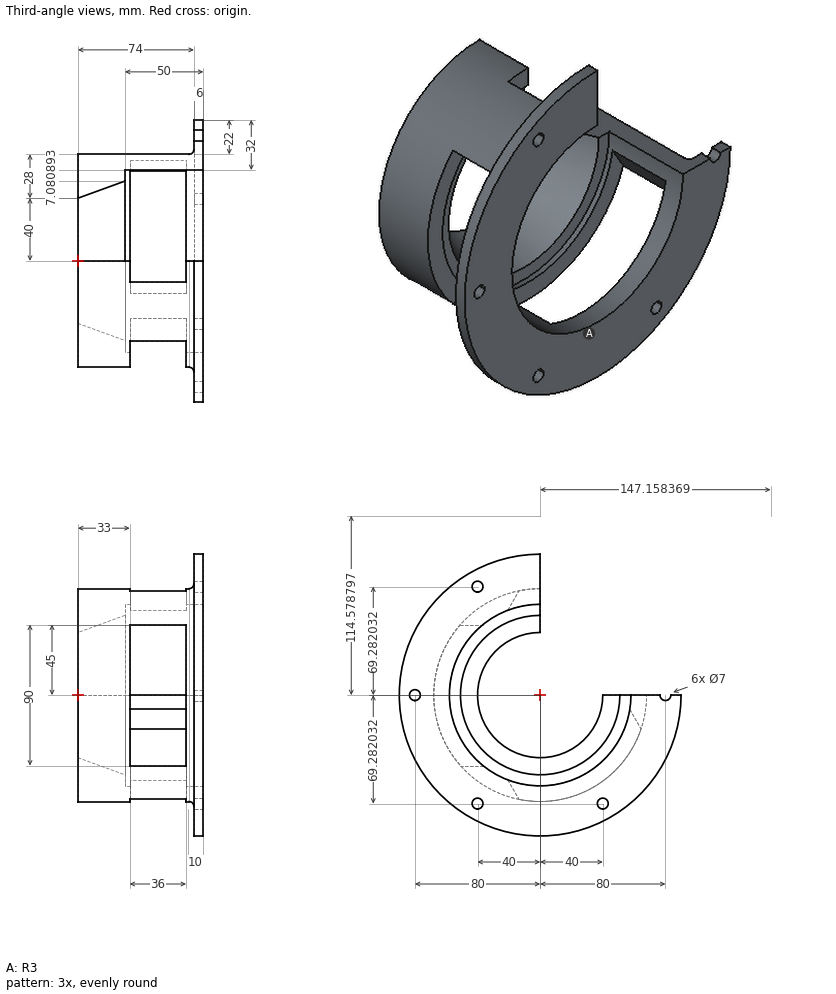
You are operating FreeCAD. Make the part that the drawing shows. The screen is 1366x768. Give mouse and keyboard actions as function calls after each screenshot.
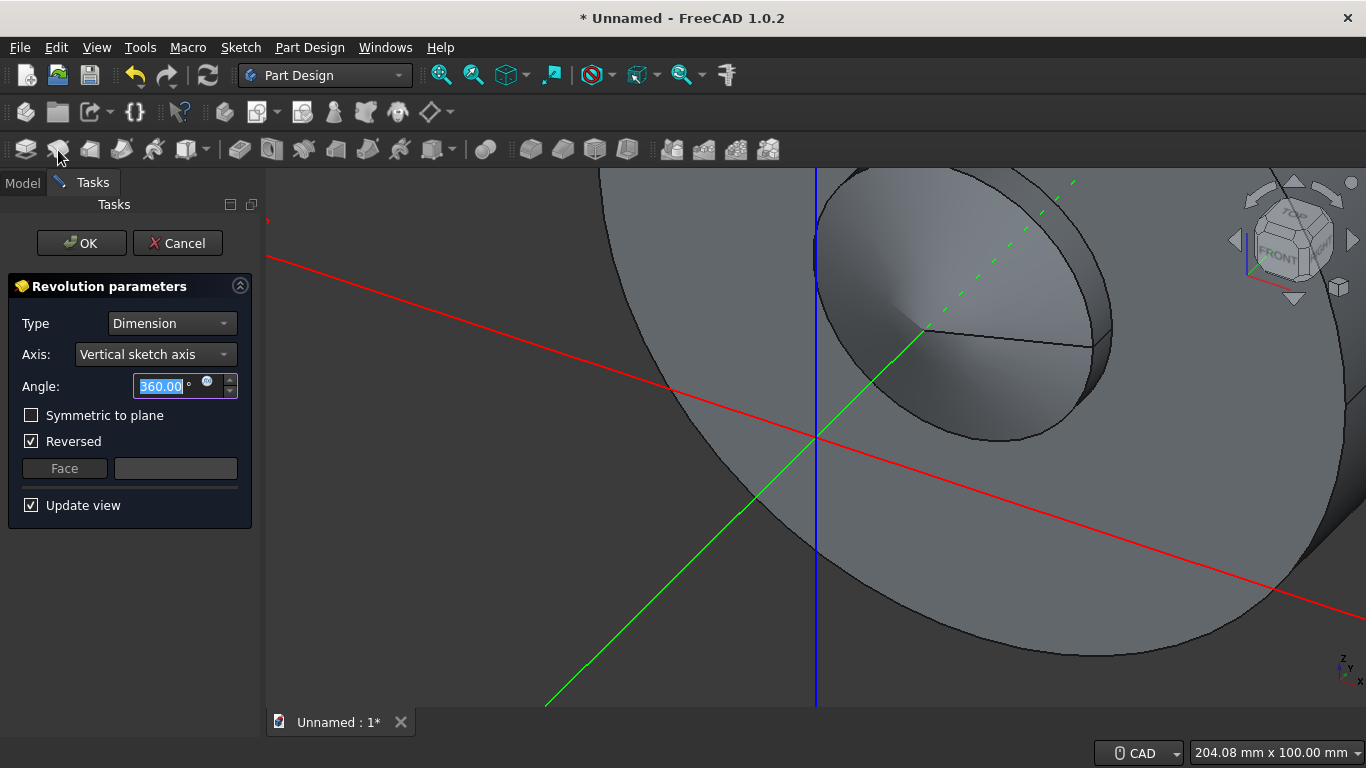
click(156, 354)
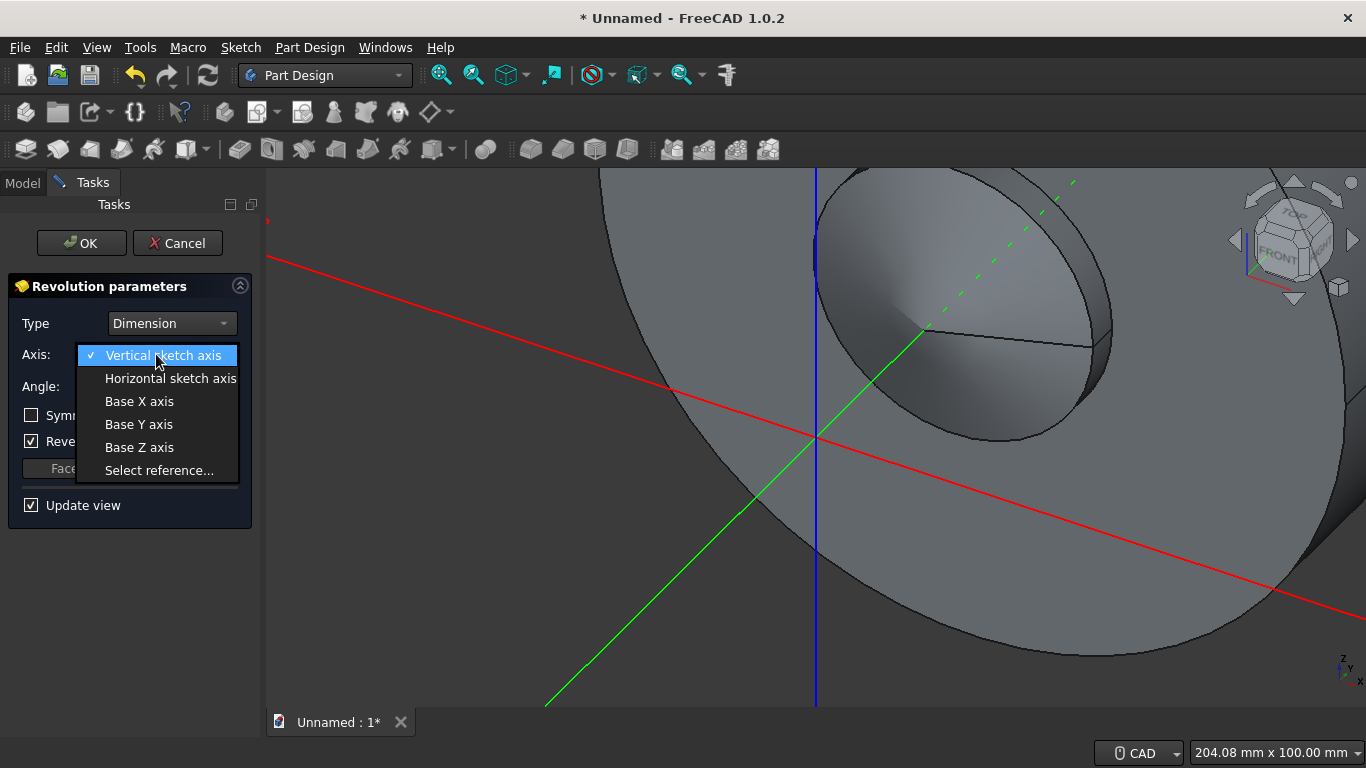
click(156, 378)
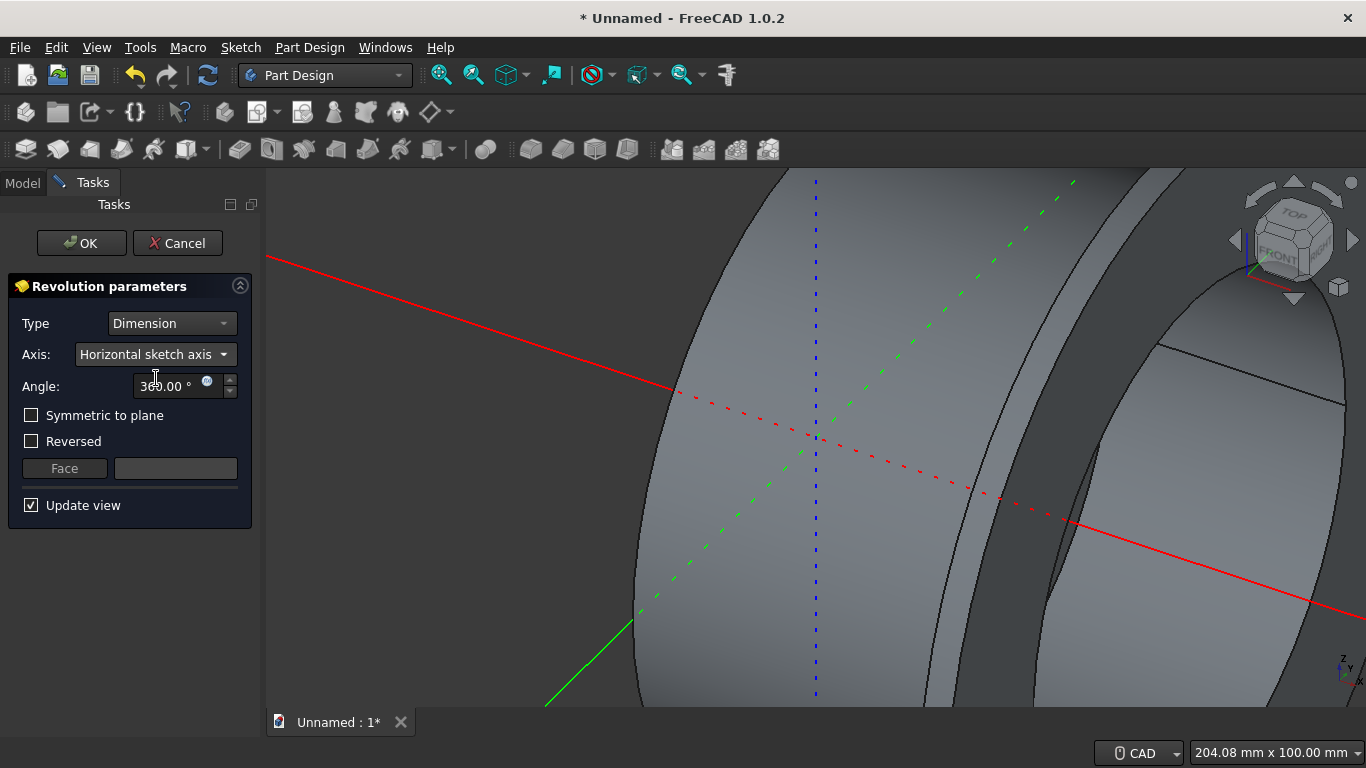
click(82, 243)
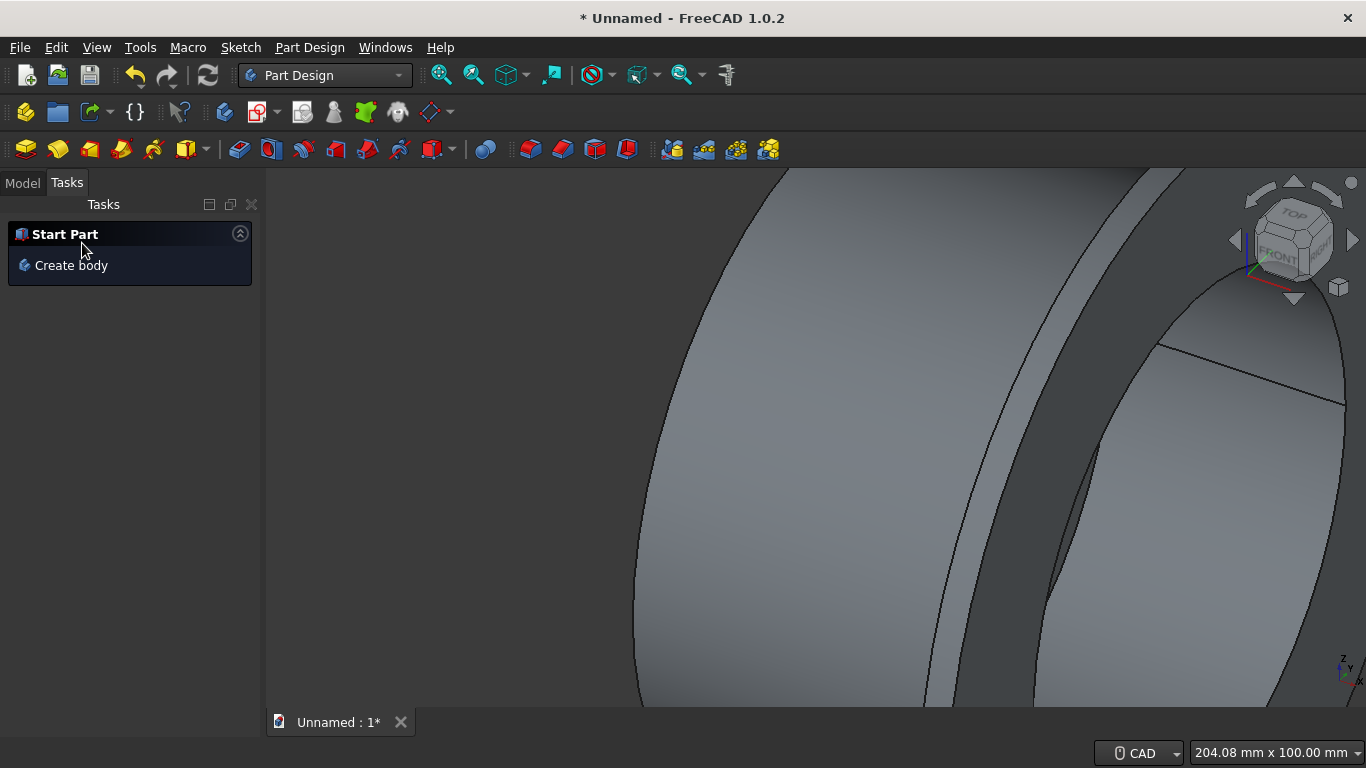
key(v)
key(f)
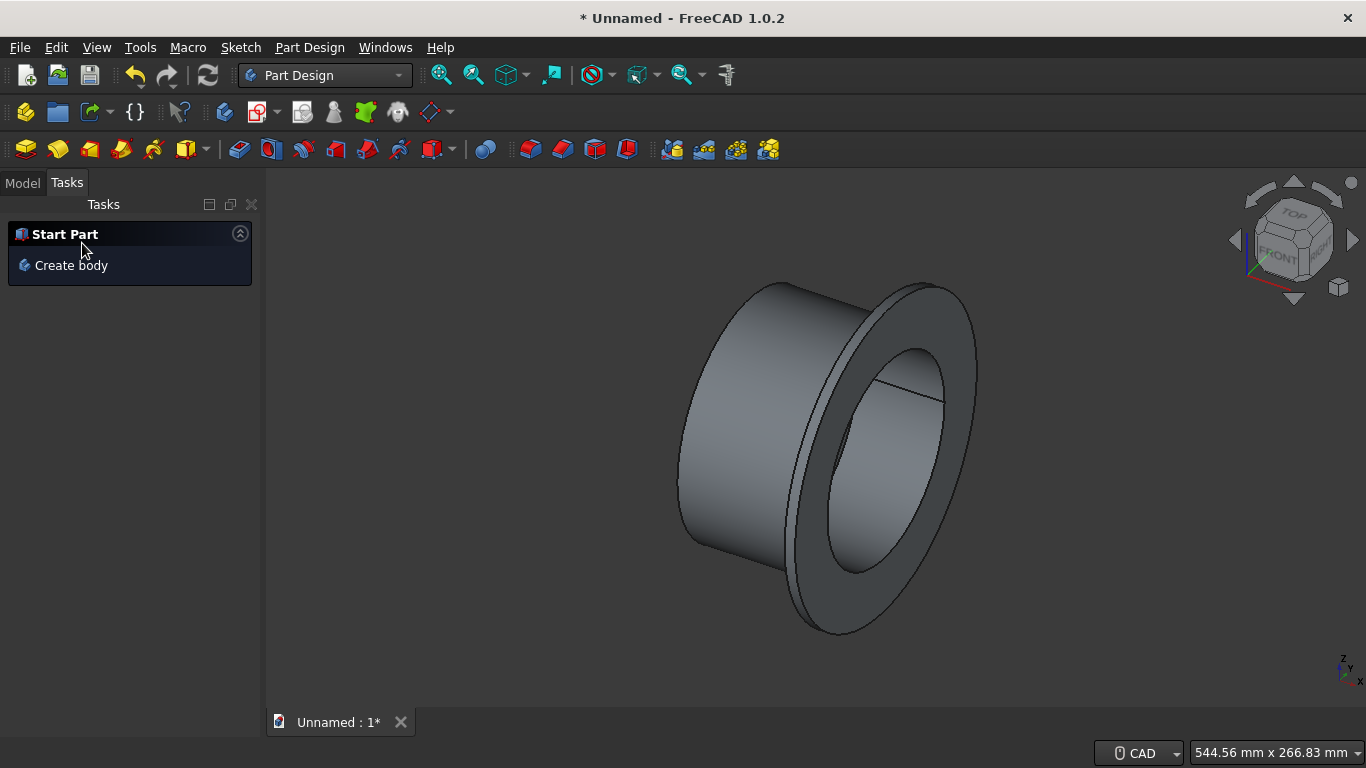
click(938, 493)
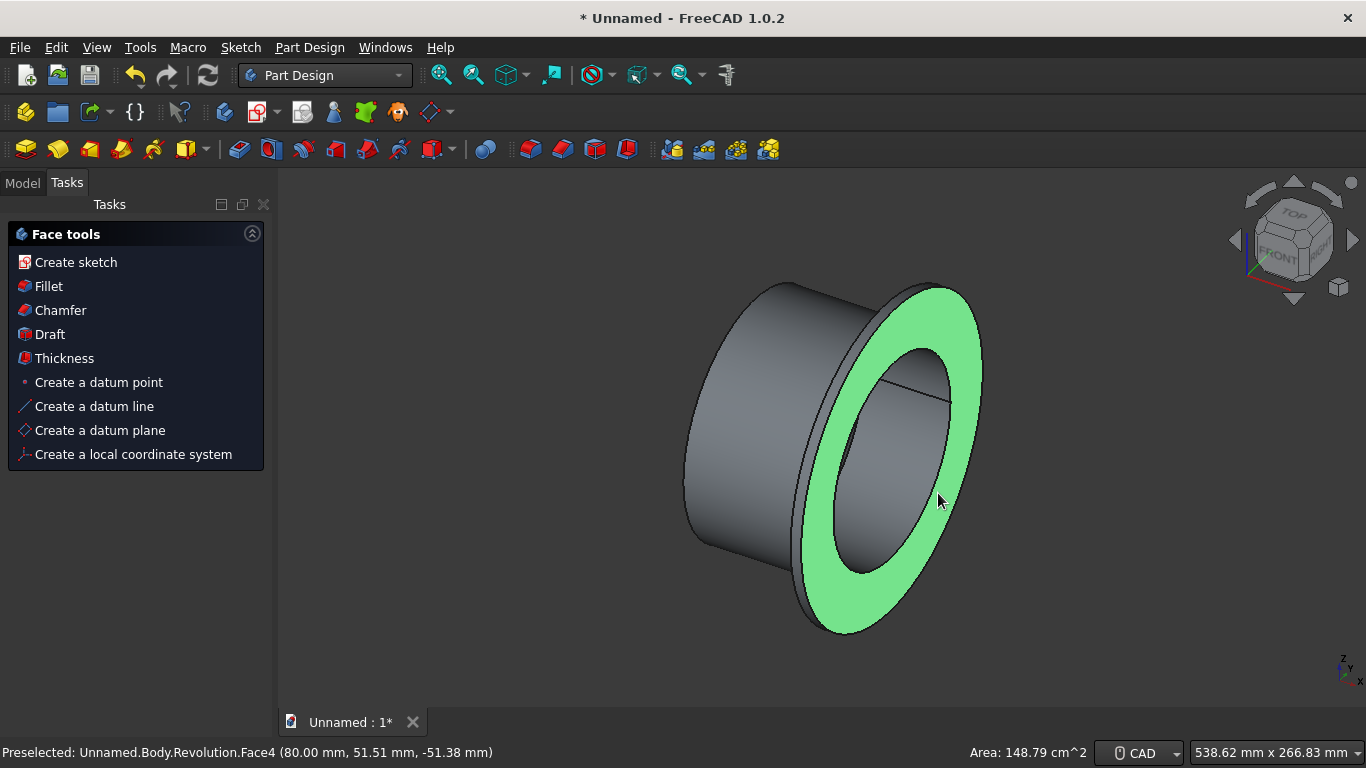
click(258, 112)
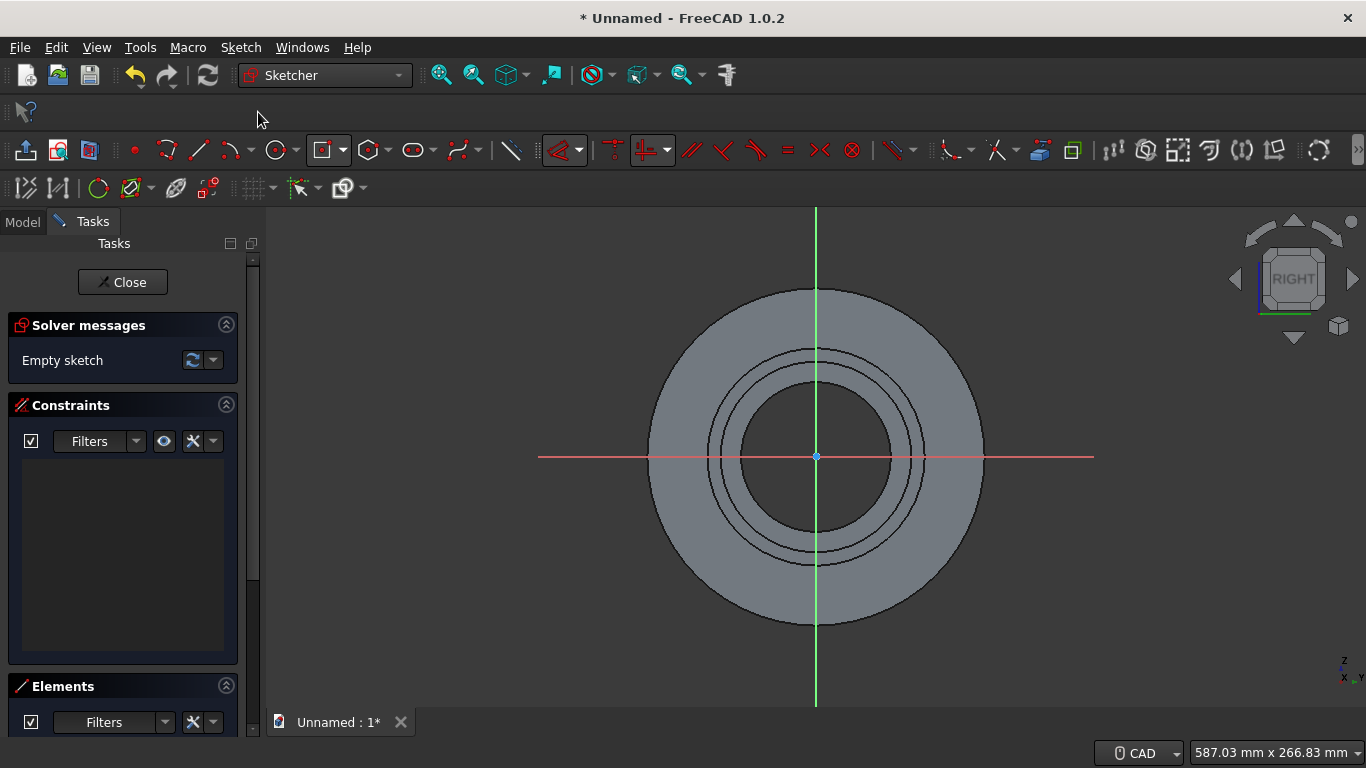
key(g)
key(c)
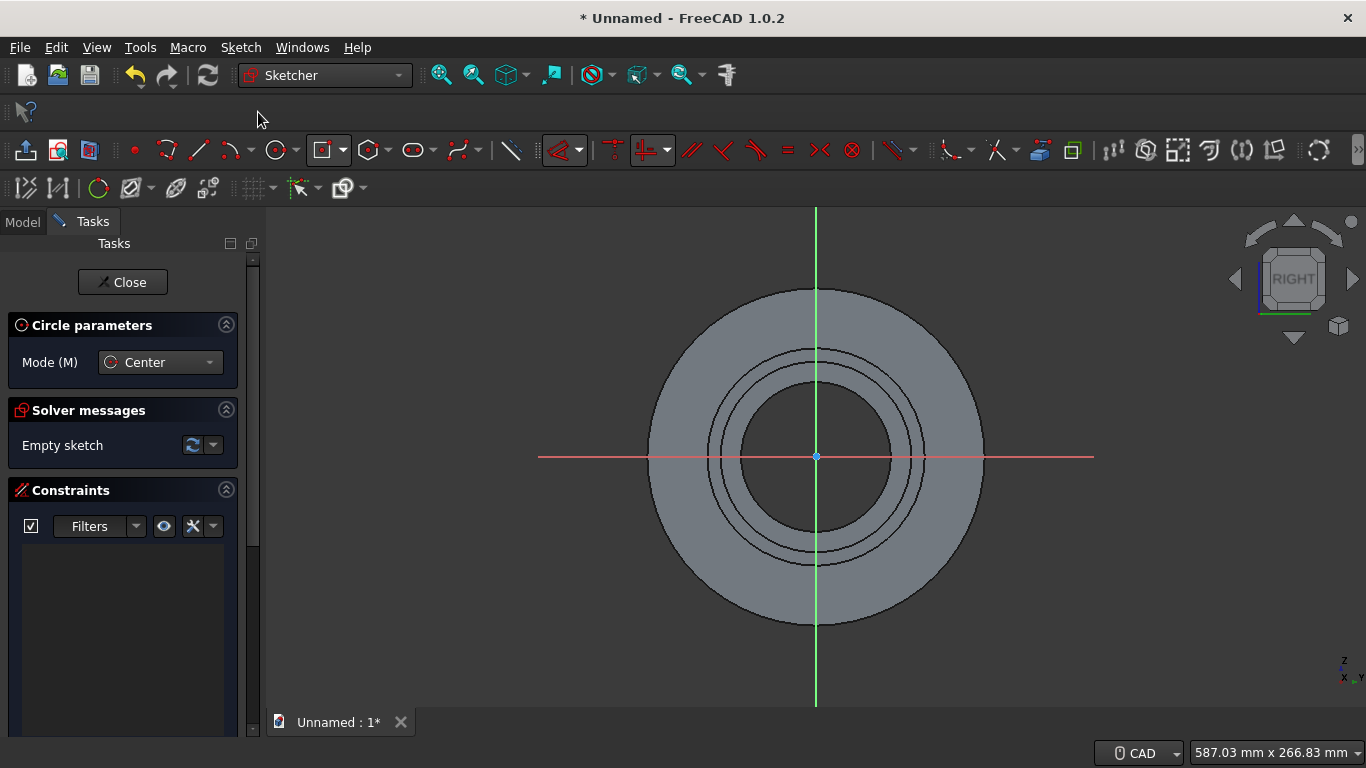
scroll(966, 457, up, 7)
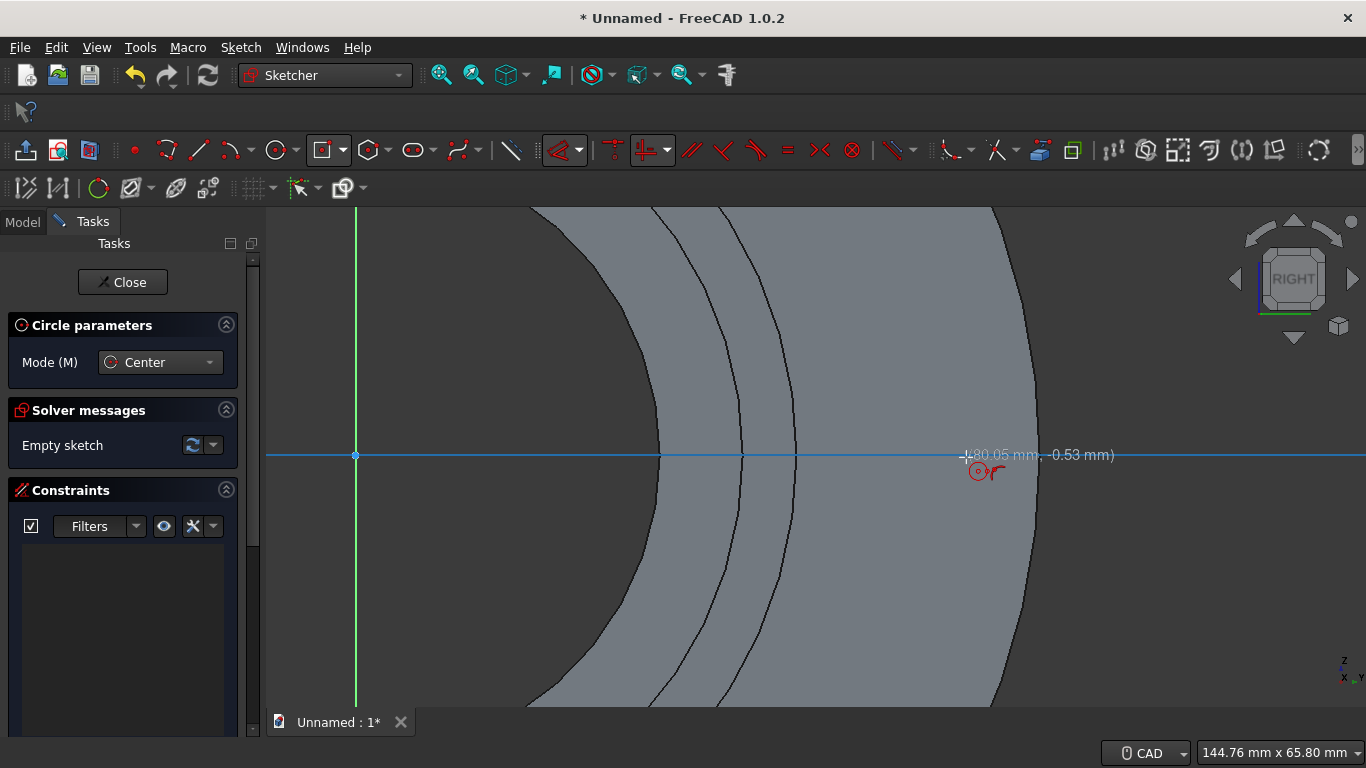
scroll(916, 458, down, 6)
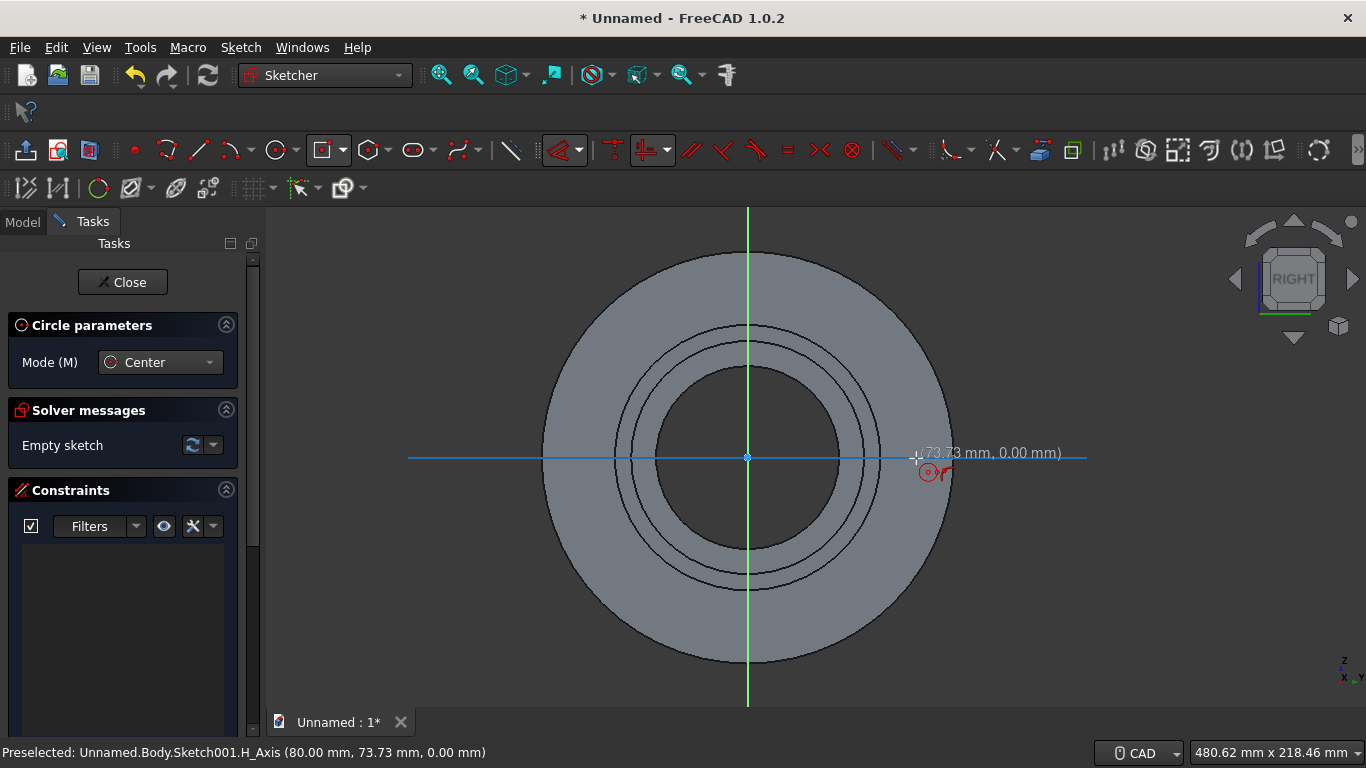
click(931, 458)